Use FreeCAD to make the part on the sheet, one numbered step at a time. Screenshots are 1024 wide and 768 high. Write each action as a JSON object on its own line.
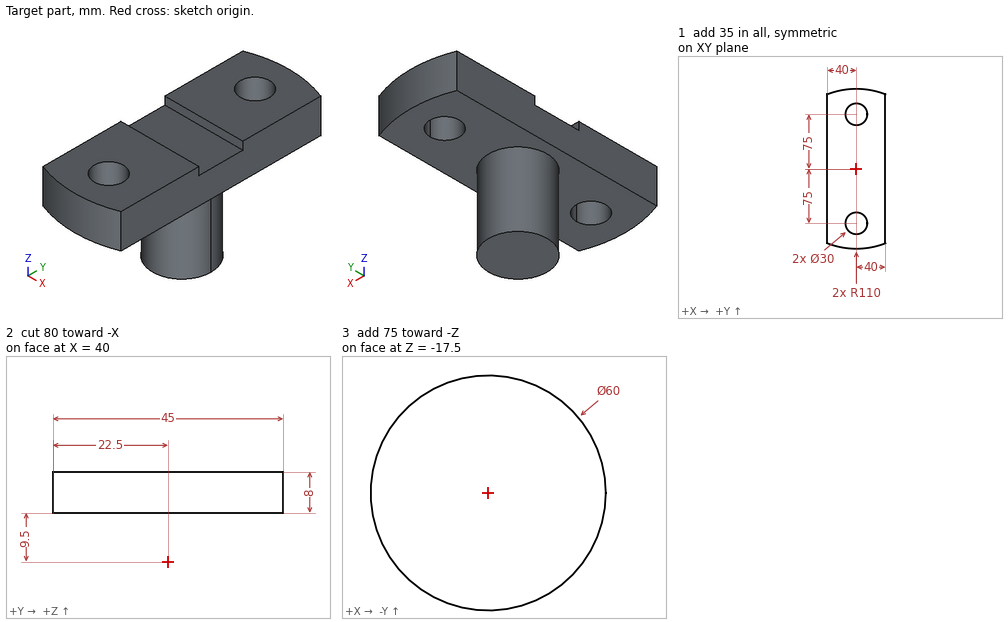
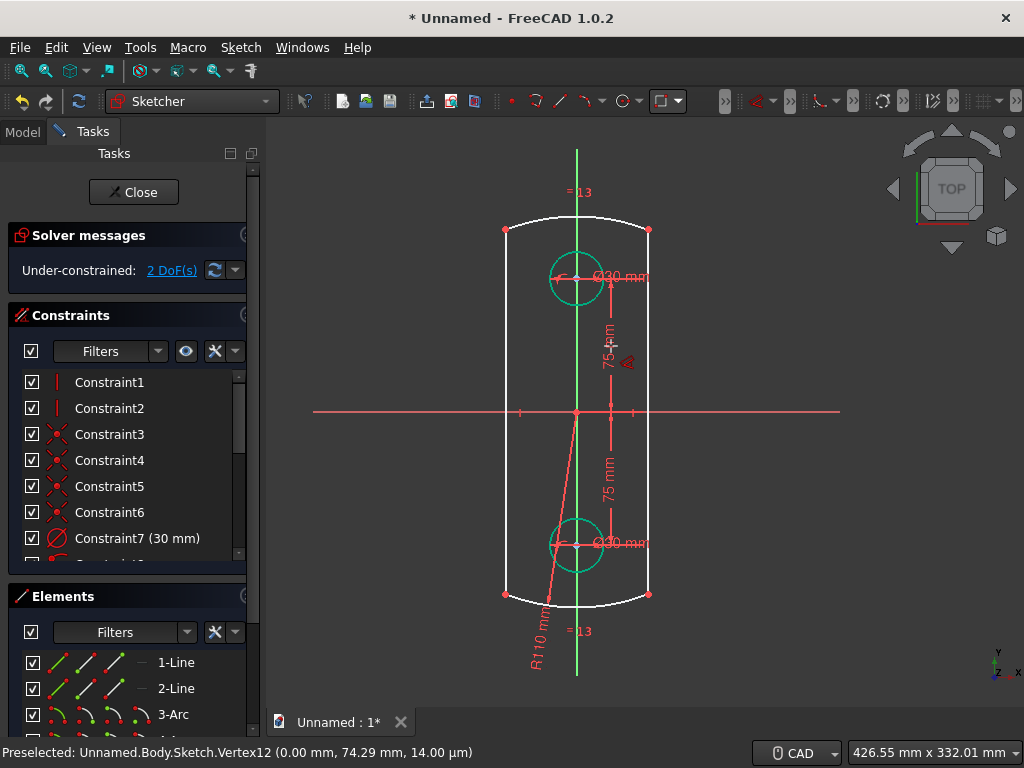
{"action": "left_click", "coordinate": [506, 230]}
{"action": "left_click", "coordinate": [541, 196]}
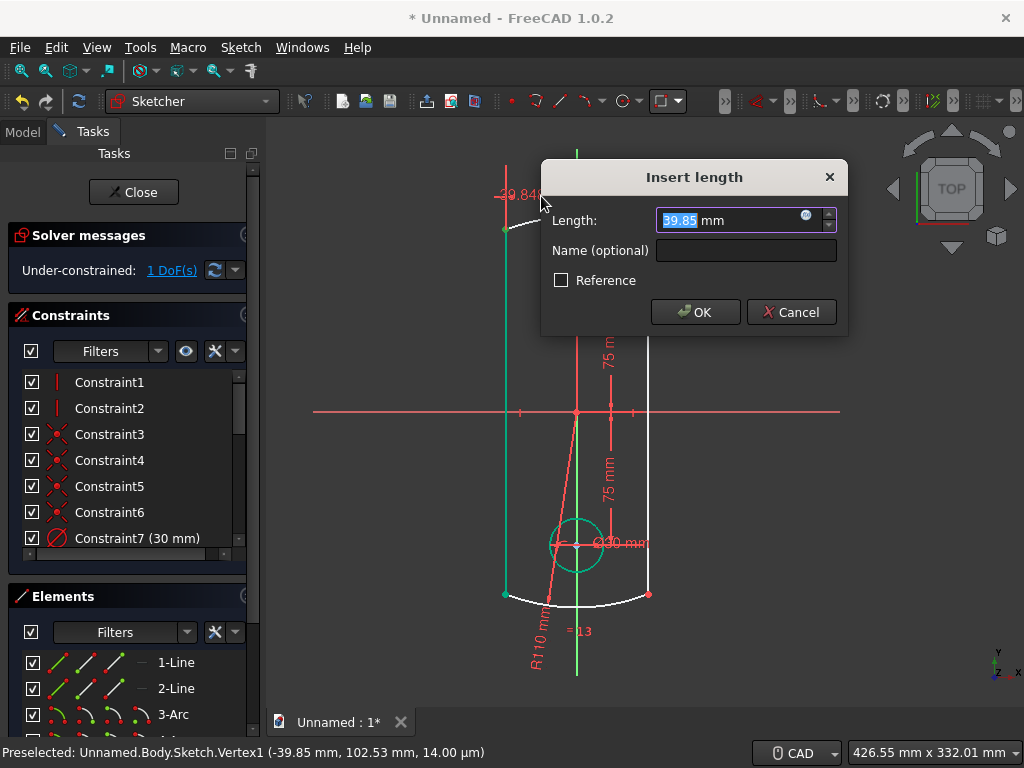
{"action": "type", "text": "40"}
{"action": "key", "text": "Return"}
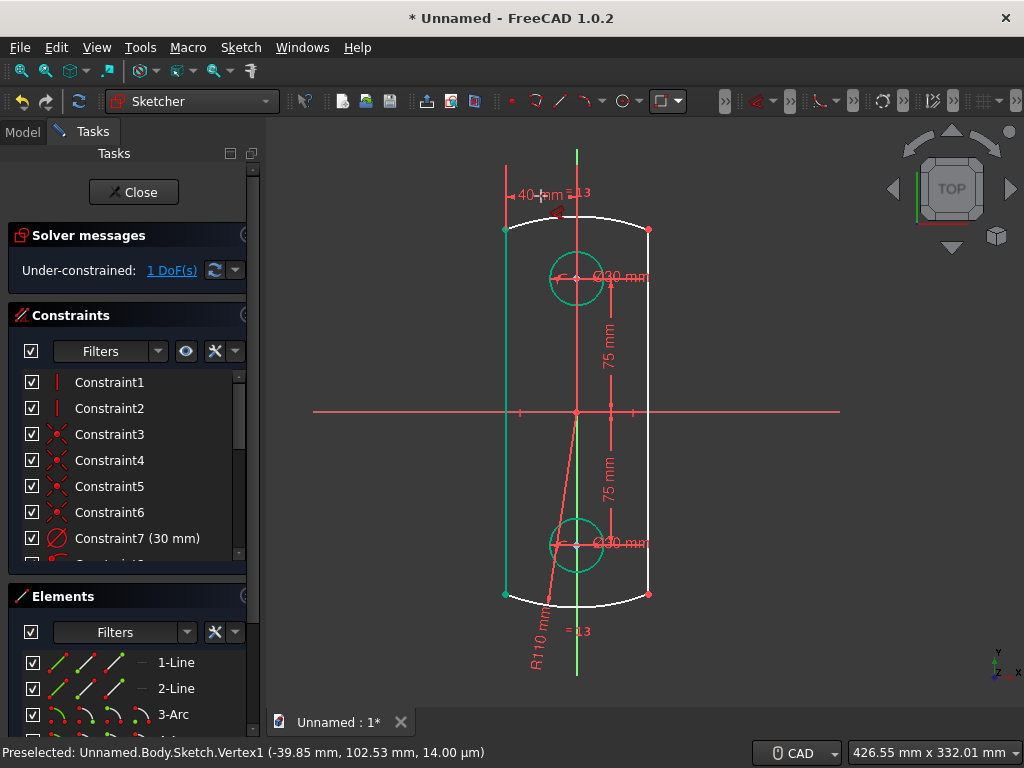
{"action": "left_click", "coordinate": [648, 594]}
{"action": "left_click", "coordinate": [629, 628]}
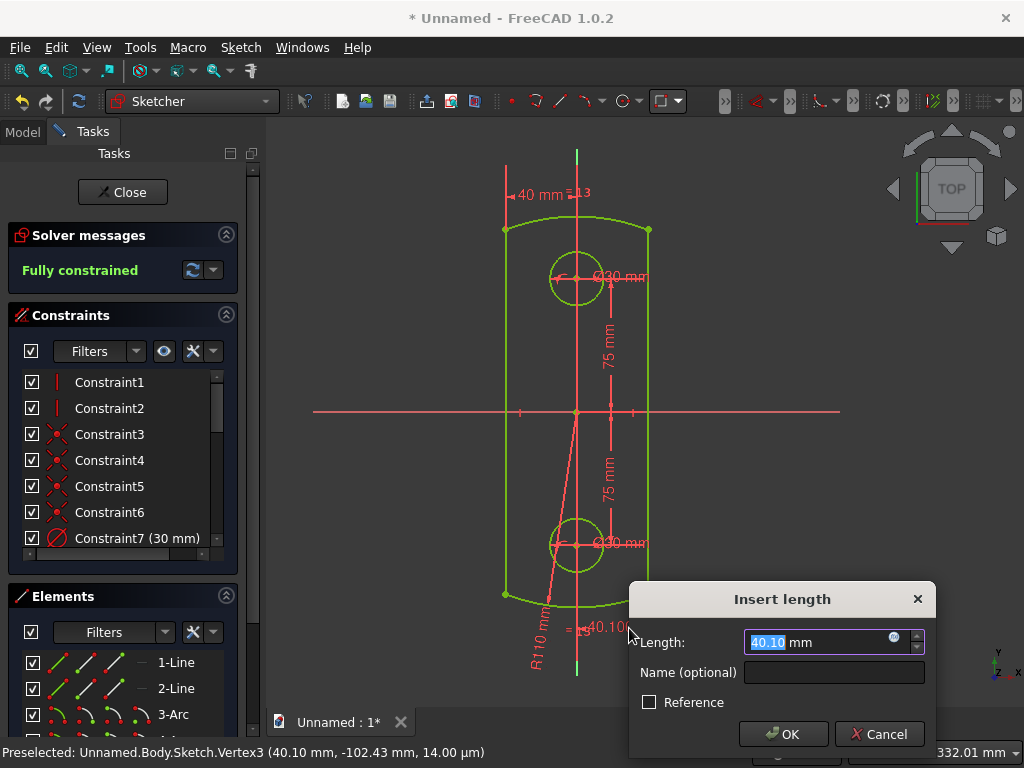
{"action": "type", "text": "40"}
{"action": "key", "text": "Return"}
{"action": "key", "text": "Escape"}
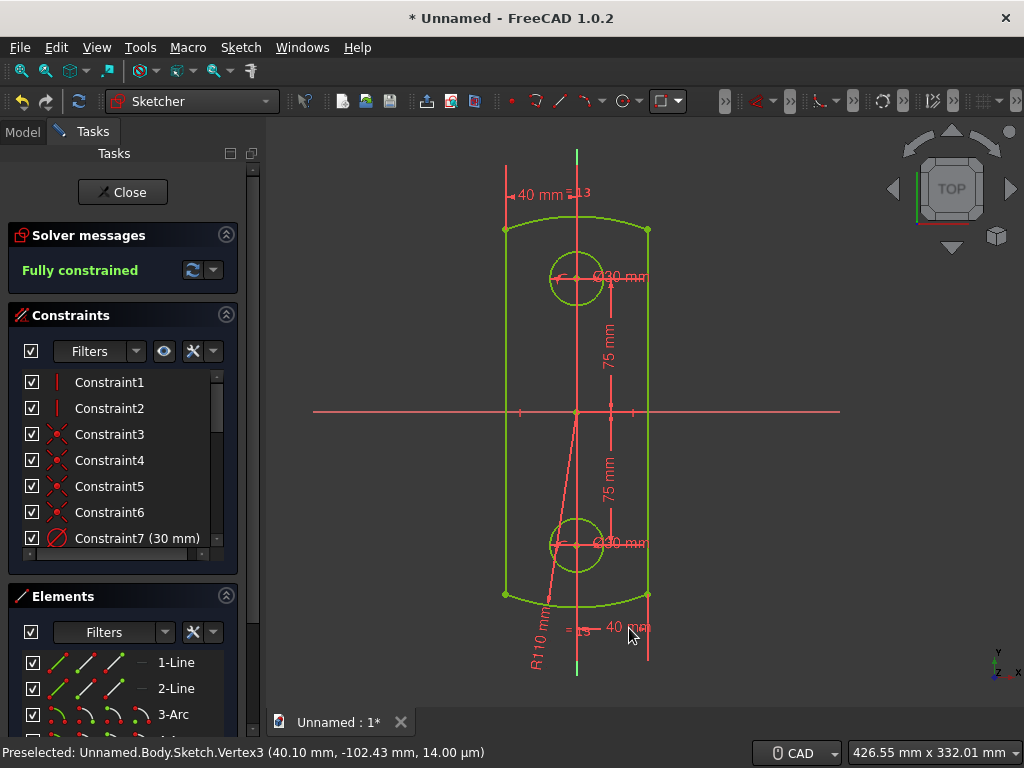
{"action": "left_click", "coordinate": [123, 192]}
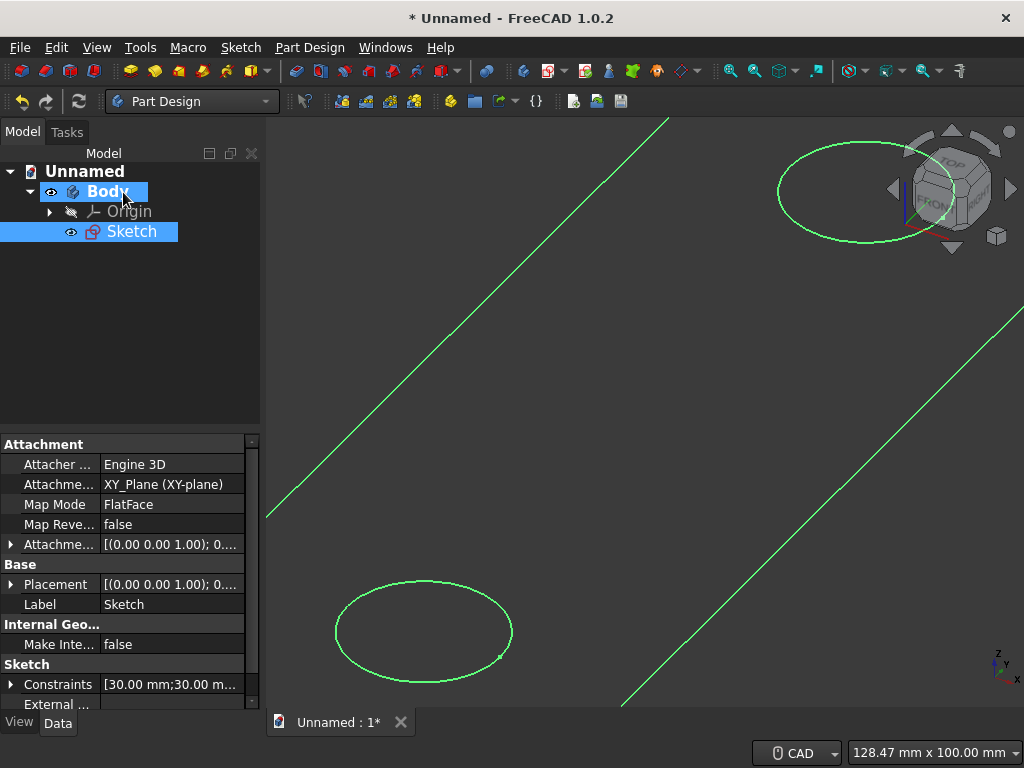
{"action": "left_click", "coordinate": [132, 72]}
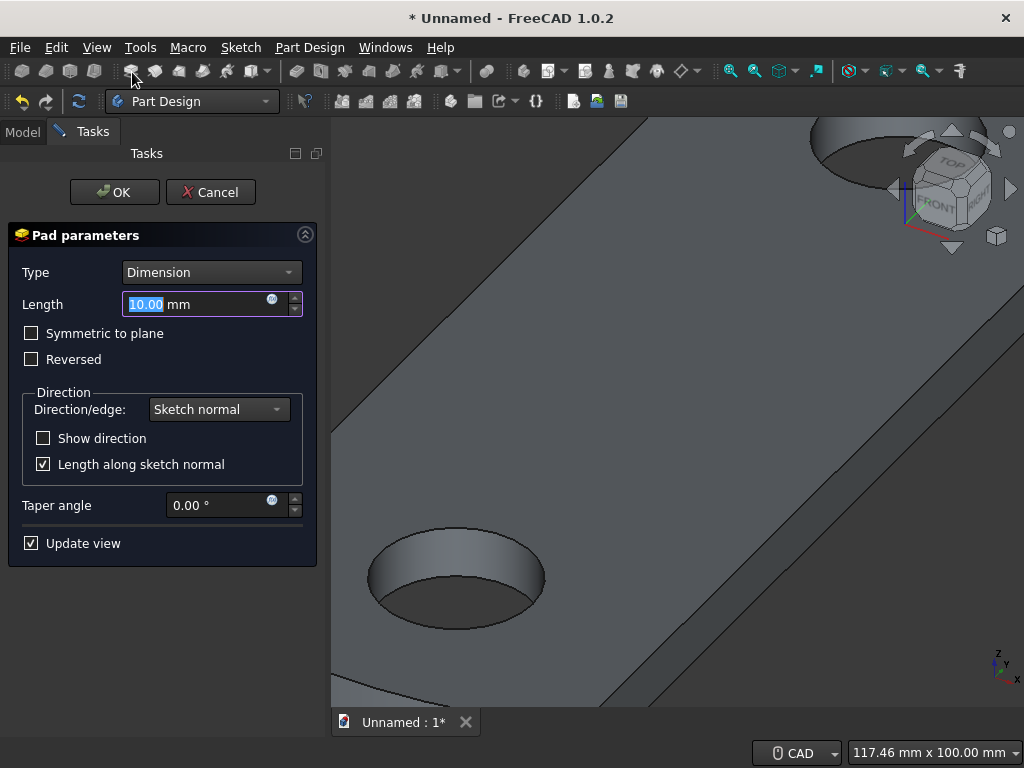
{"action": "type", "text": "35"}
{"action": "key", "text": "Tab"}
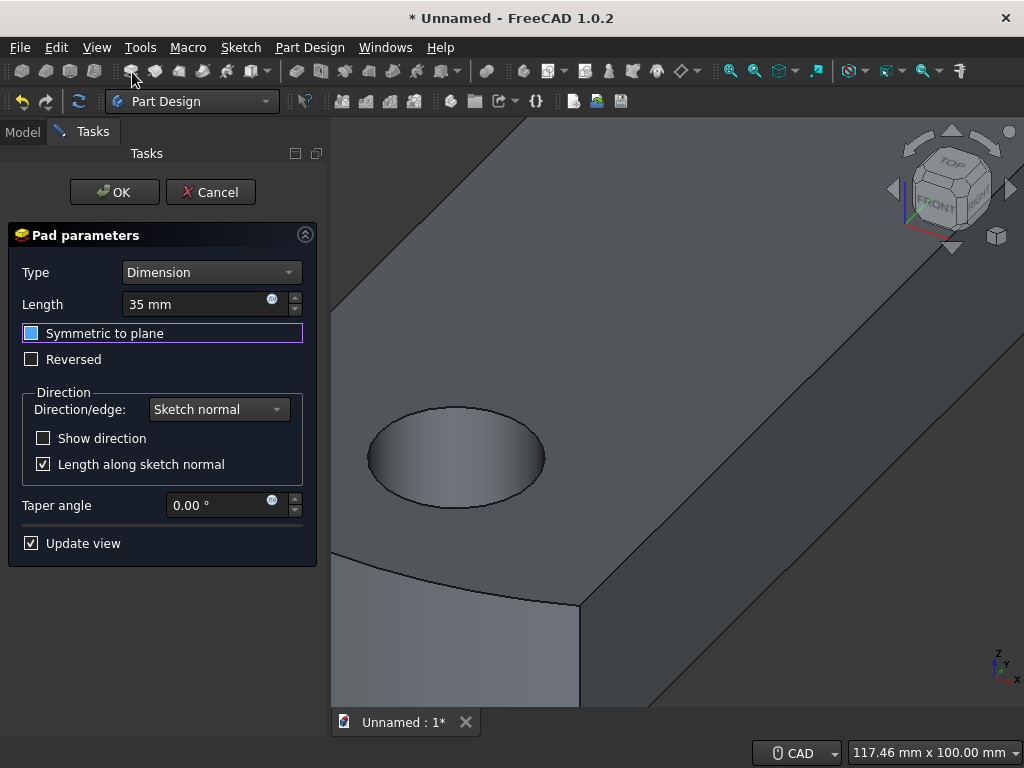
{"action": "left_click", "coordinate": [30, 333]}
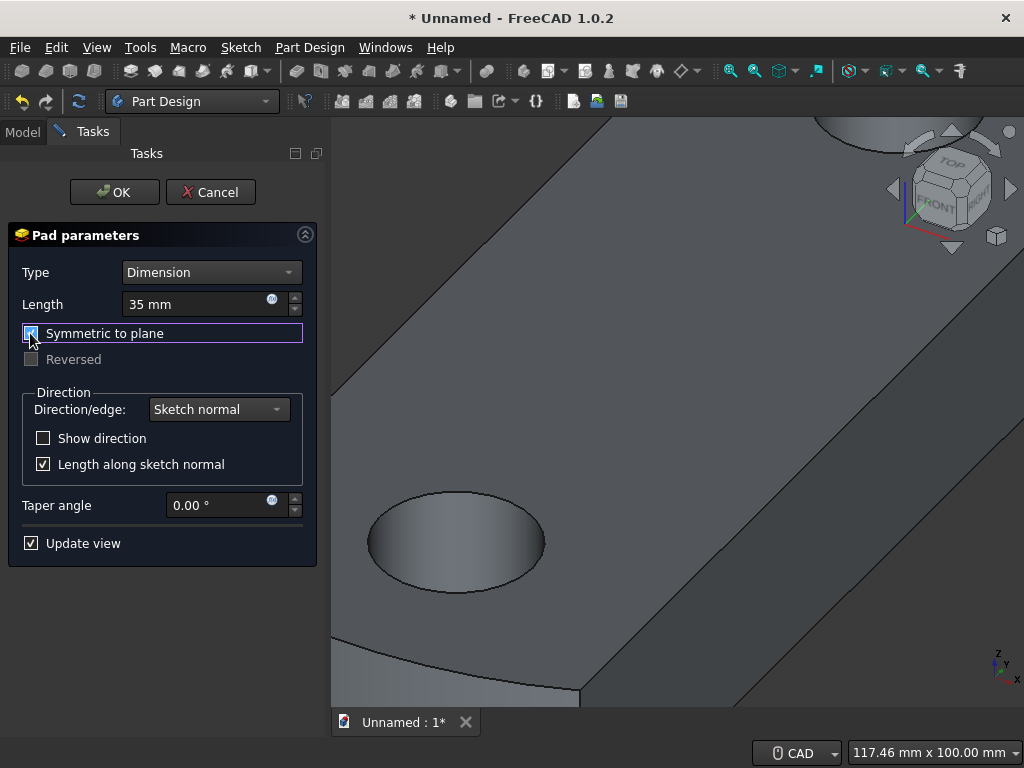
{"action": "left_click", "coordinate": [115, 192]}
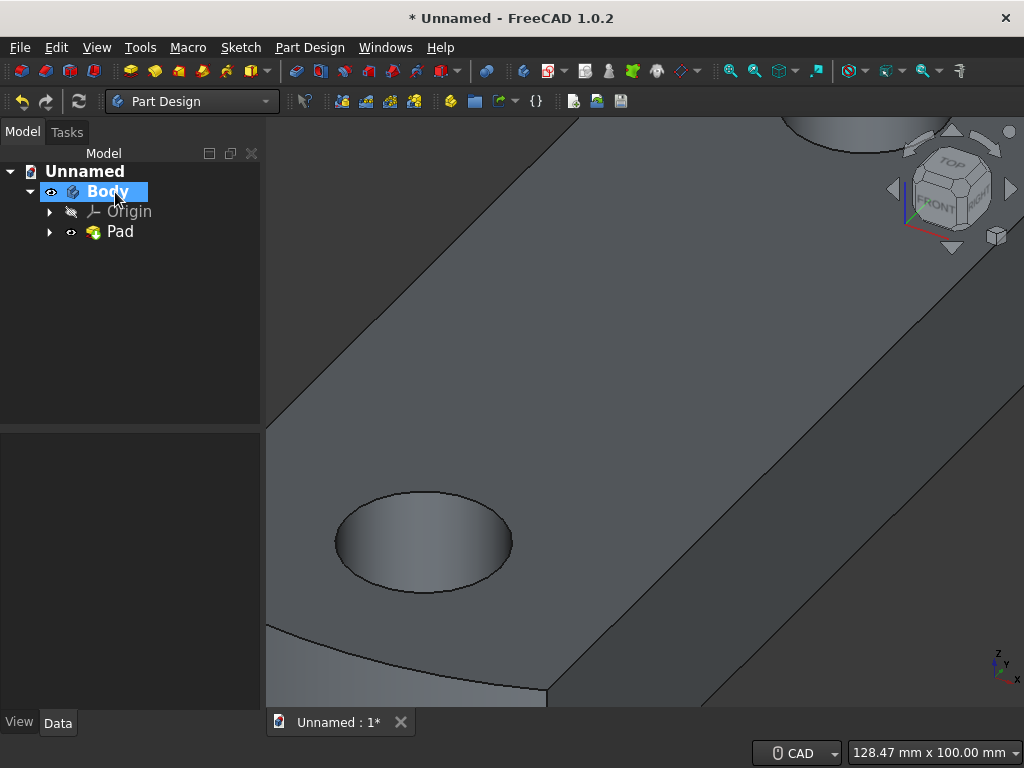
{"action": "left_click", "coordinate": [732, 72]}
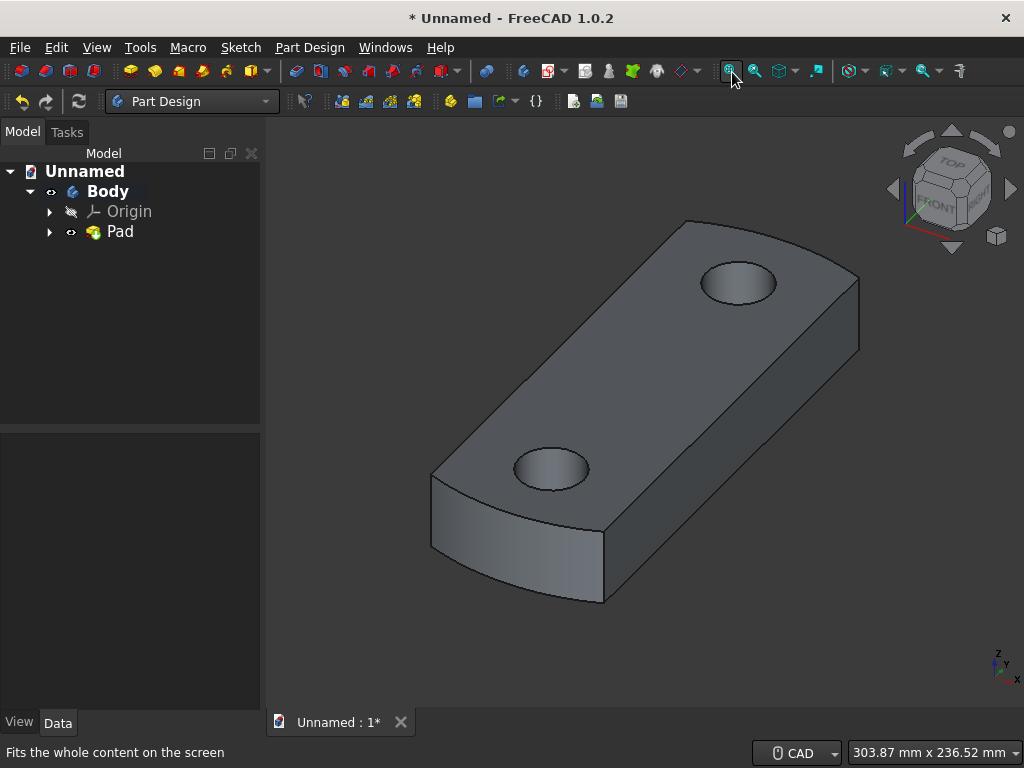
{"action": "left_click", "coordinate": [804, 367]}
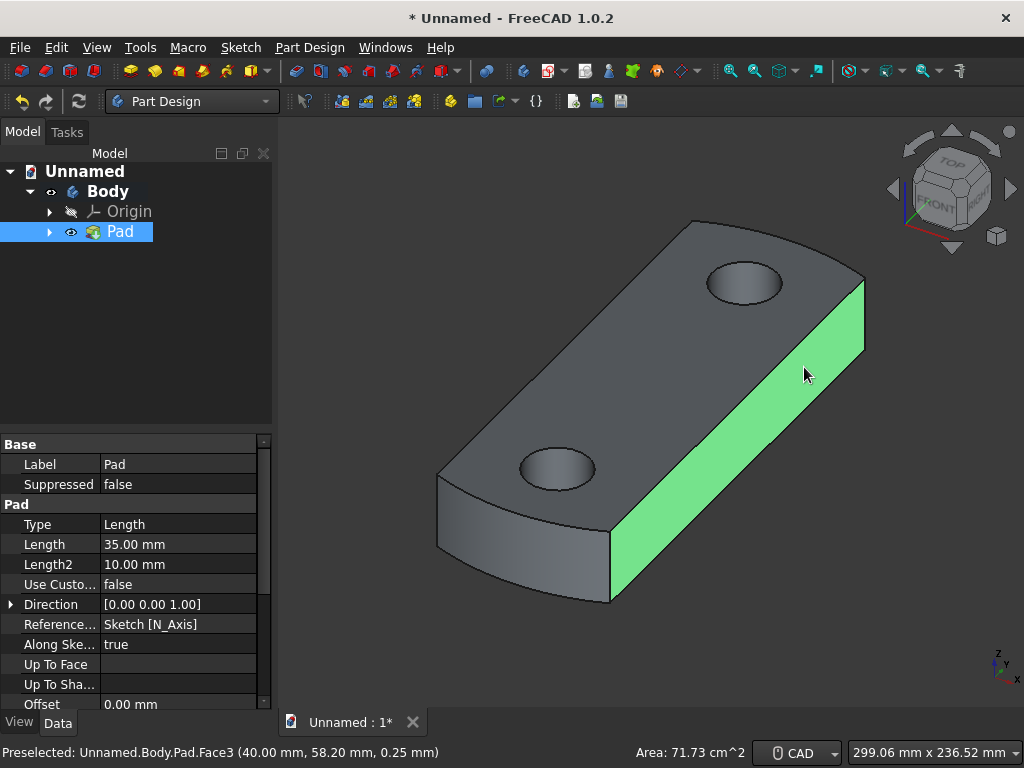
{"action": "left_click", "coordinate": [548, 72]}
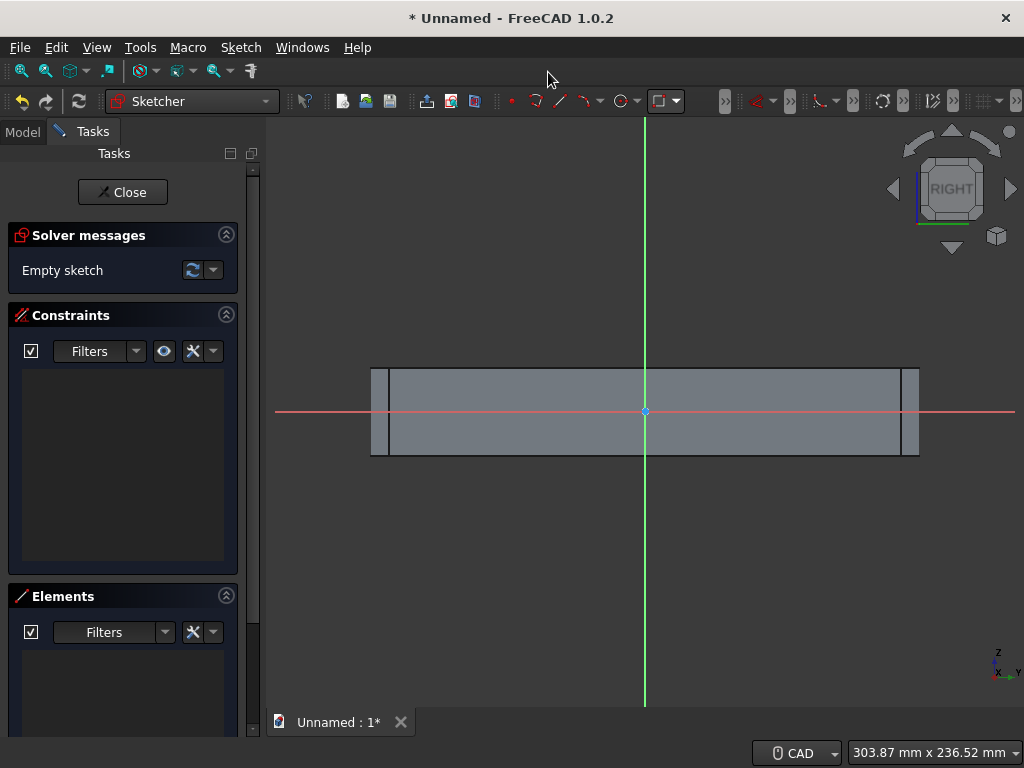
{"action": "scroll", "coordinate": [675, 381], "scroll_direction": "up", "scroll_amount": 6}